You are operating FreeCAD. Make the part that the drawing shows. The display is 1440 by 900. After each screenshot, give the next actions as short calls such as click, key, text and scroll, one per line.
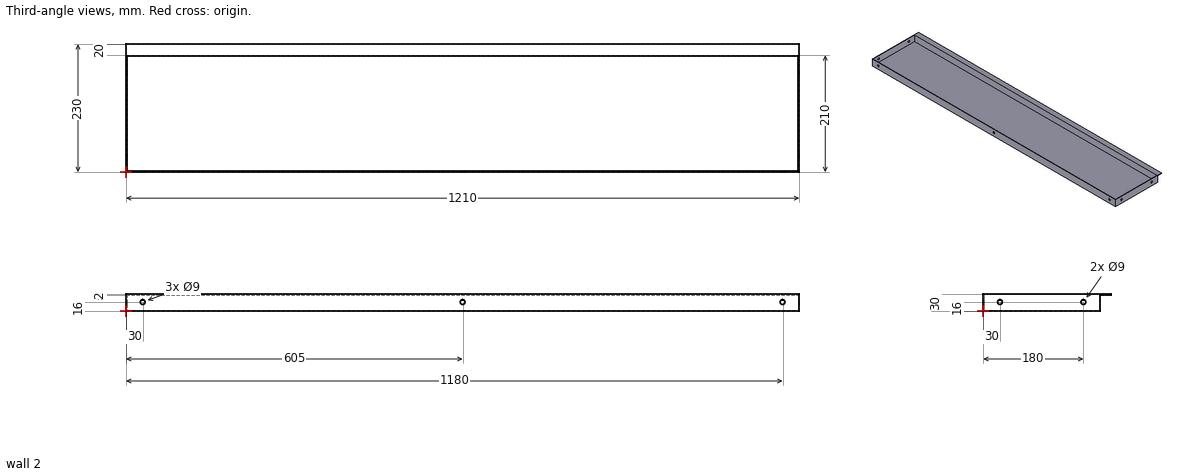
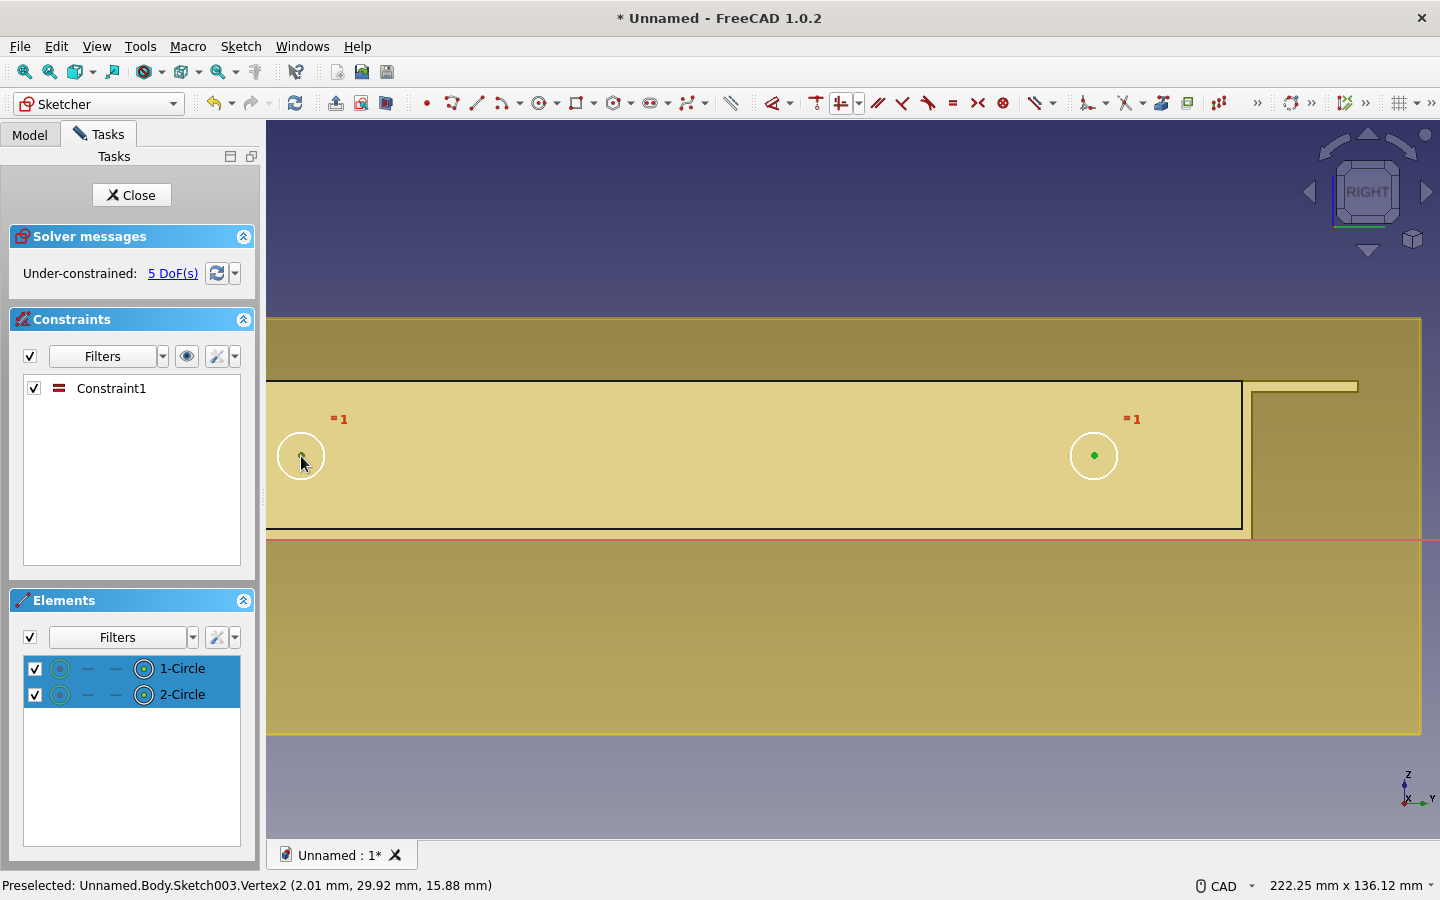
key(h)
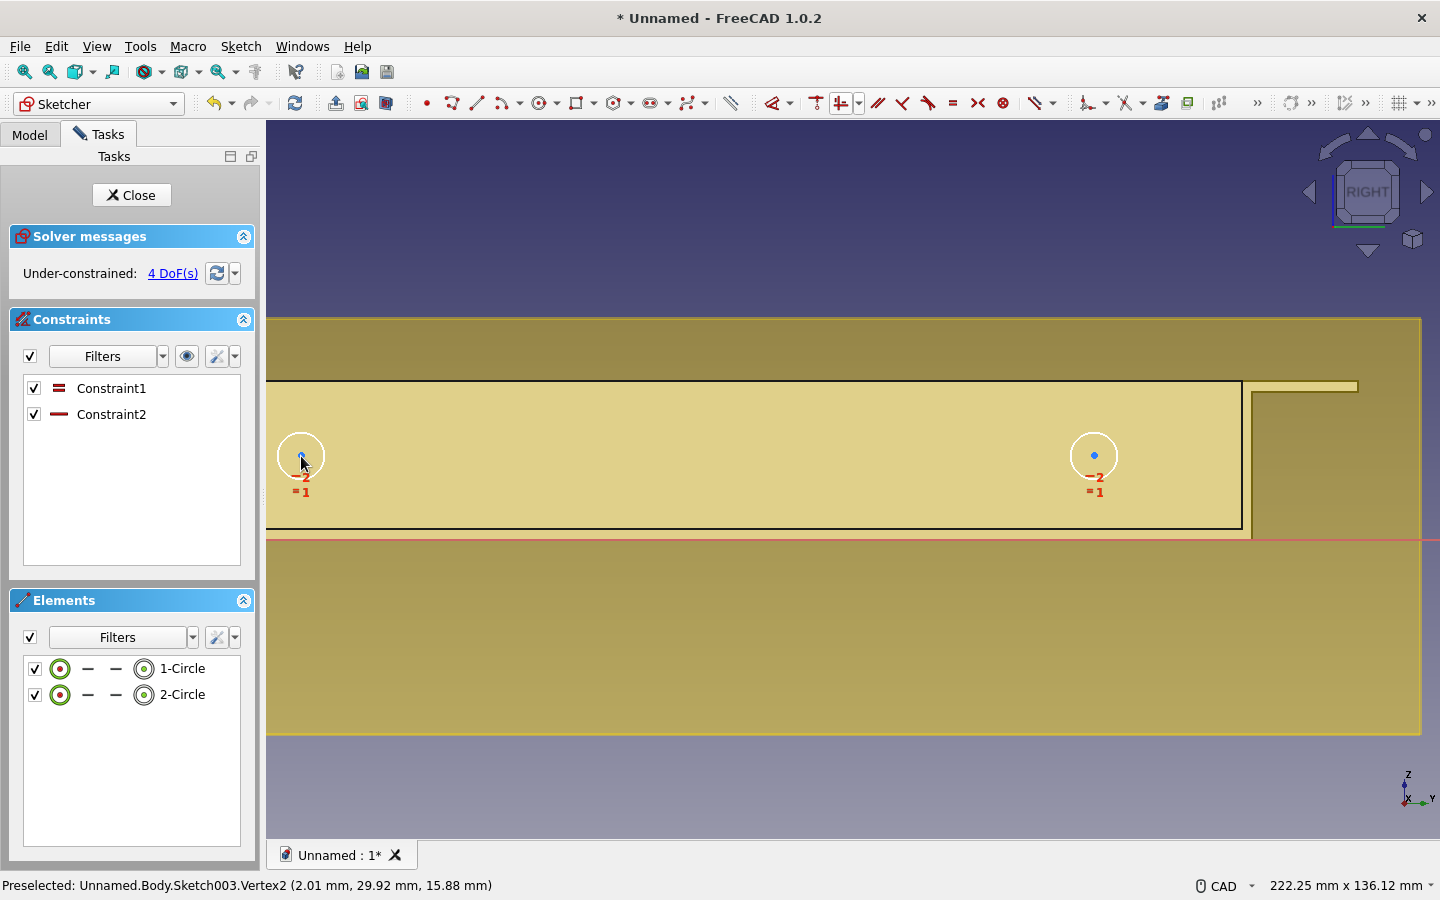
click(772, 104)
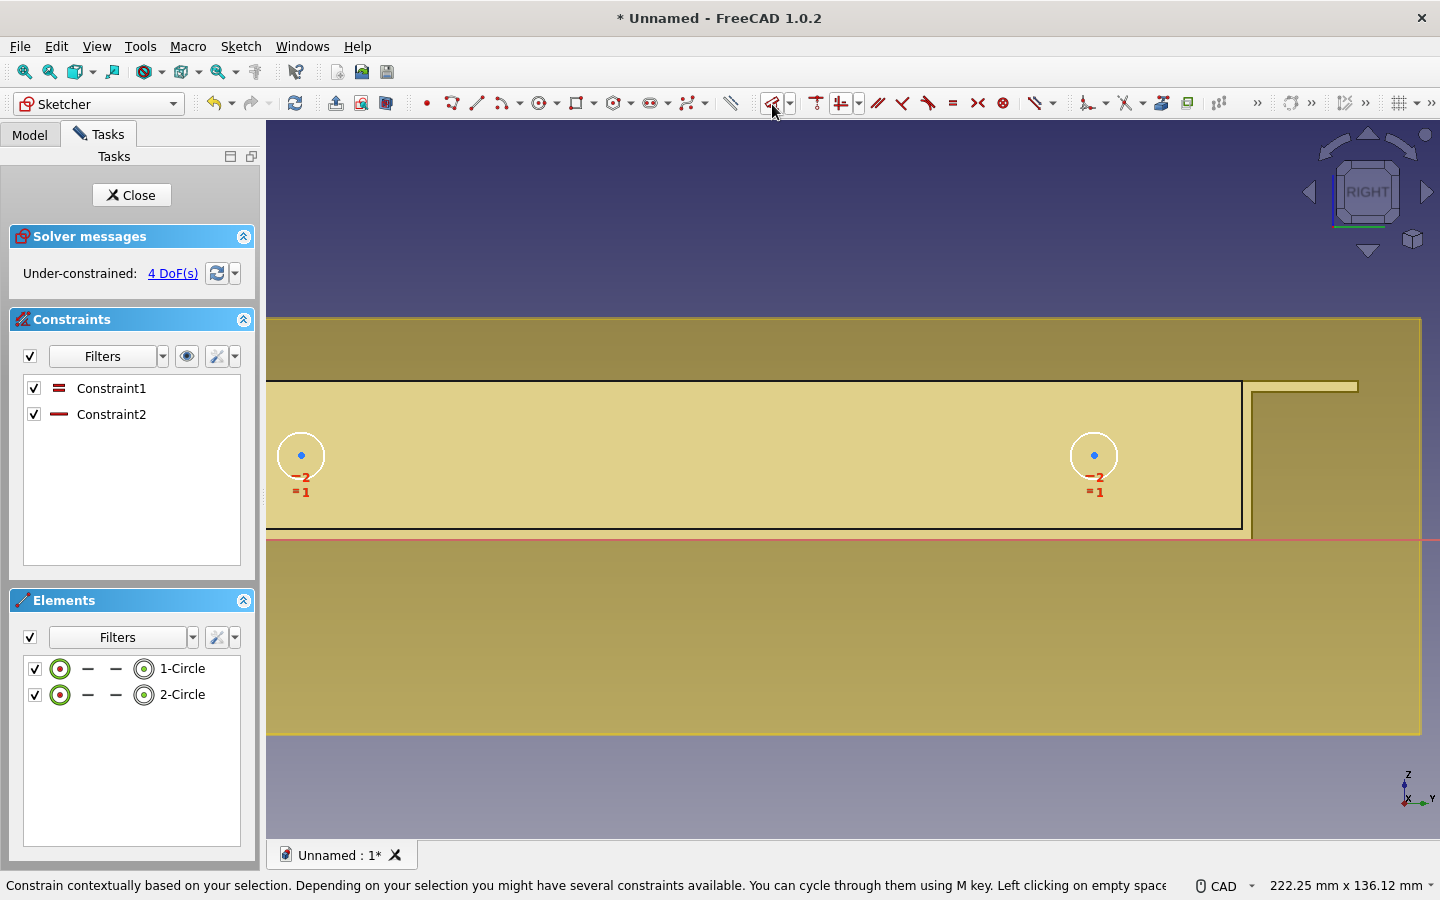
click(1110, 439)
click(1132, 416)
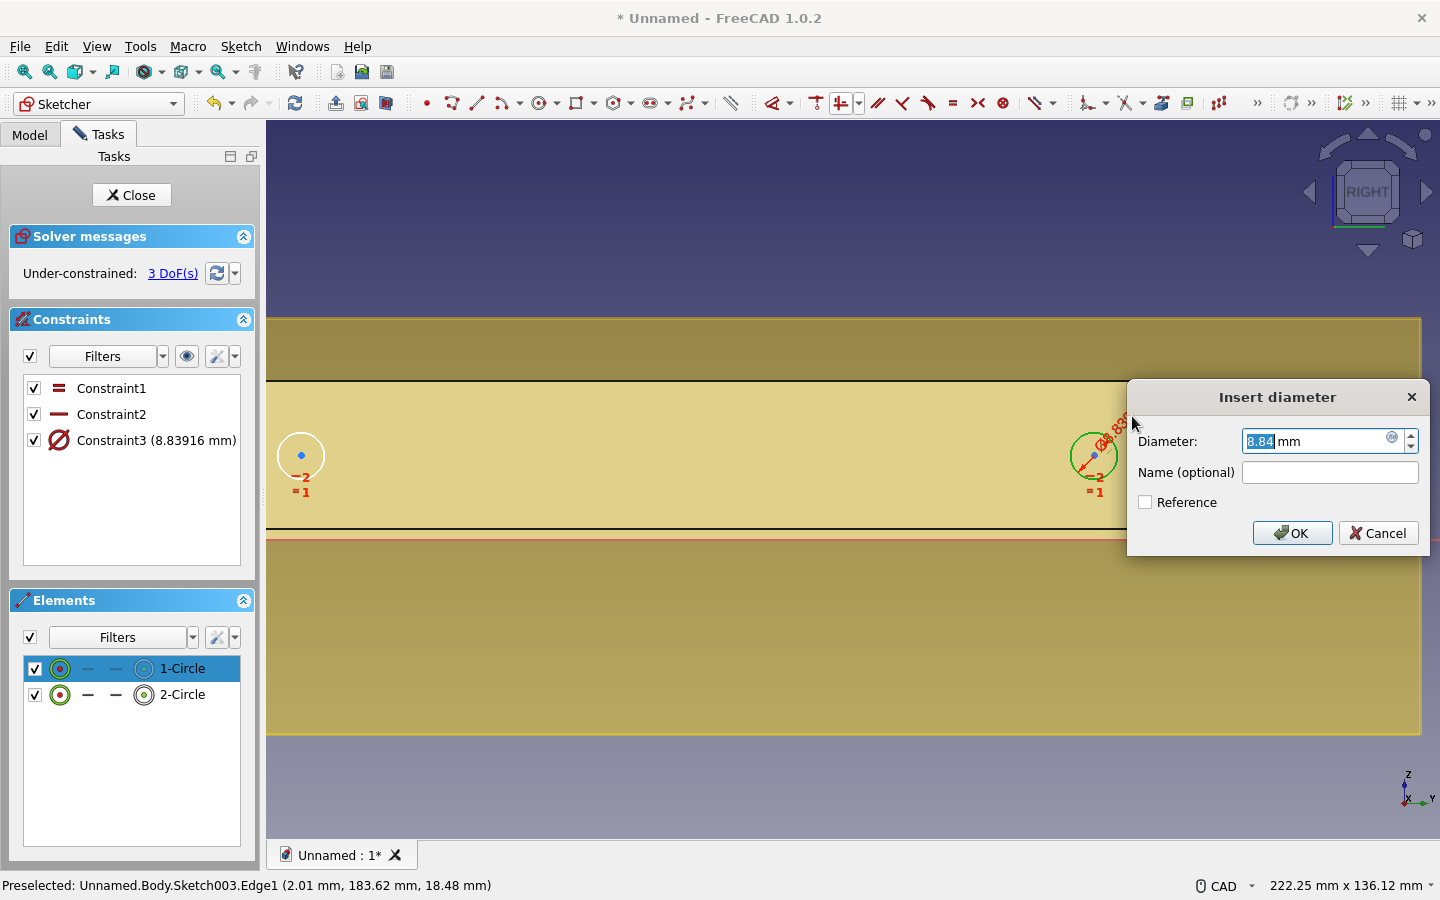
text(9)
key(Return)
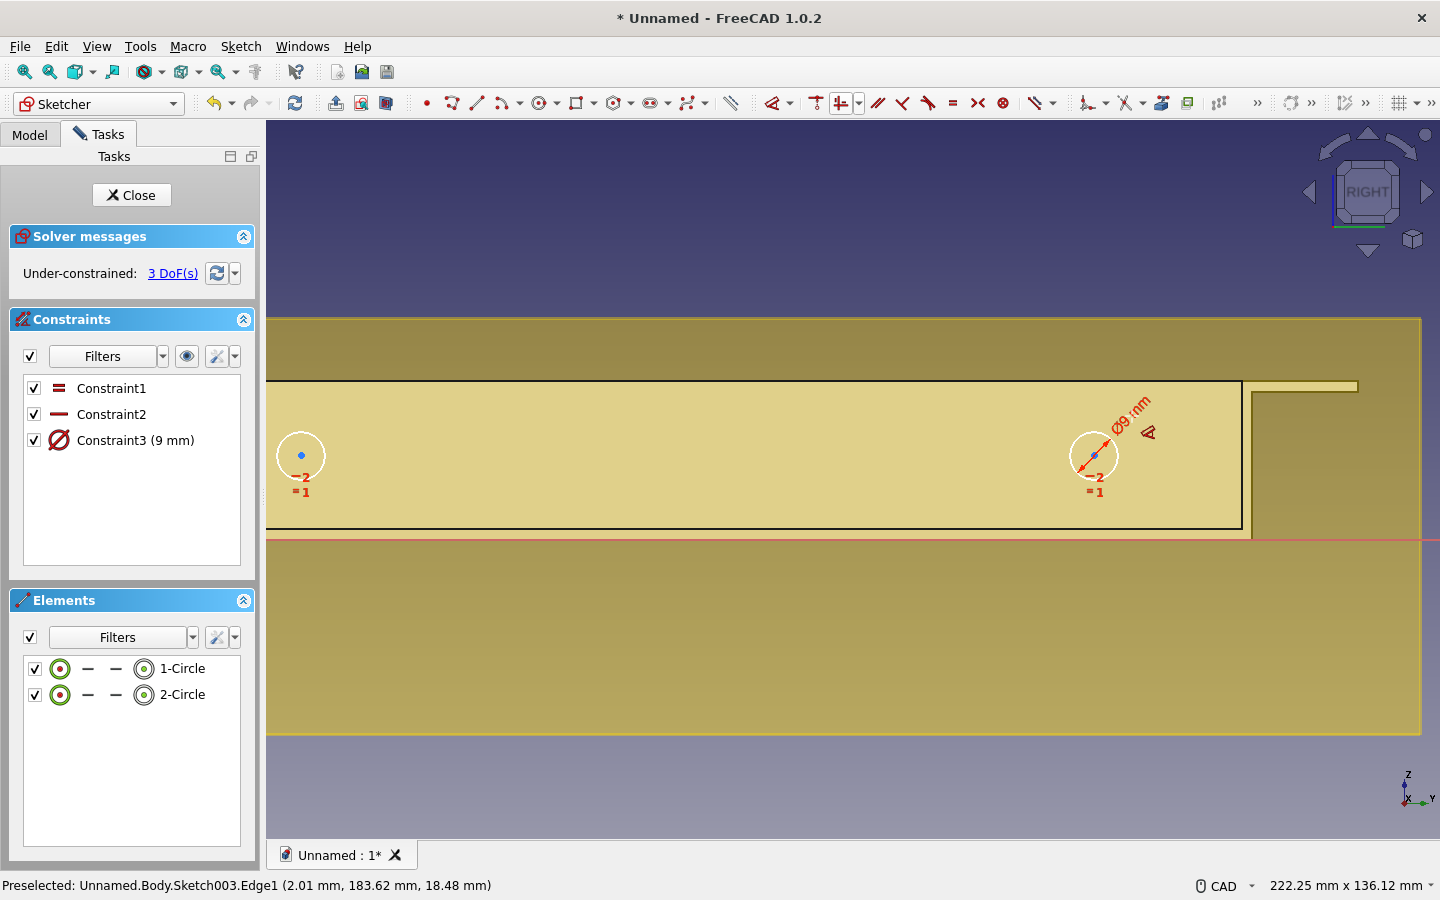
click(1094, 456)
click(1128, 498)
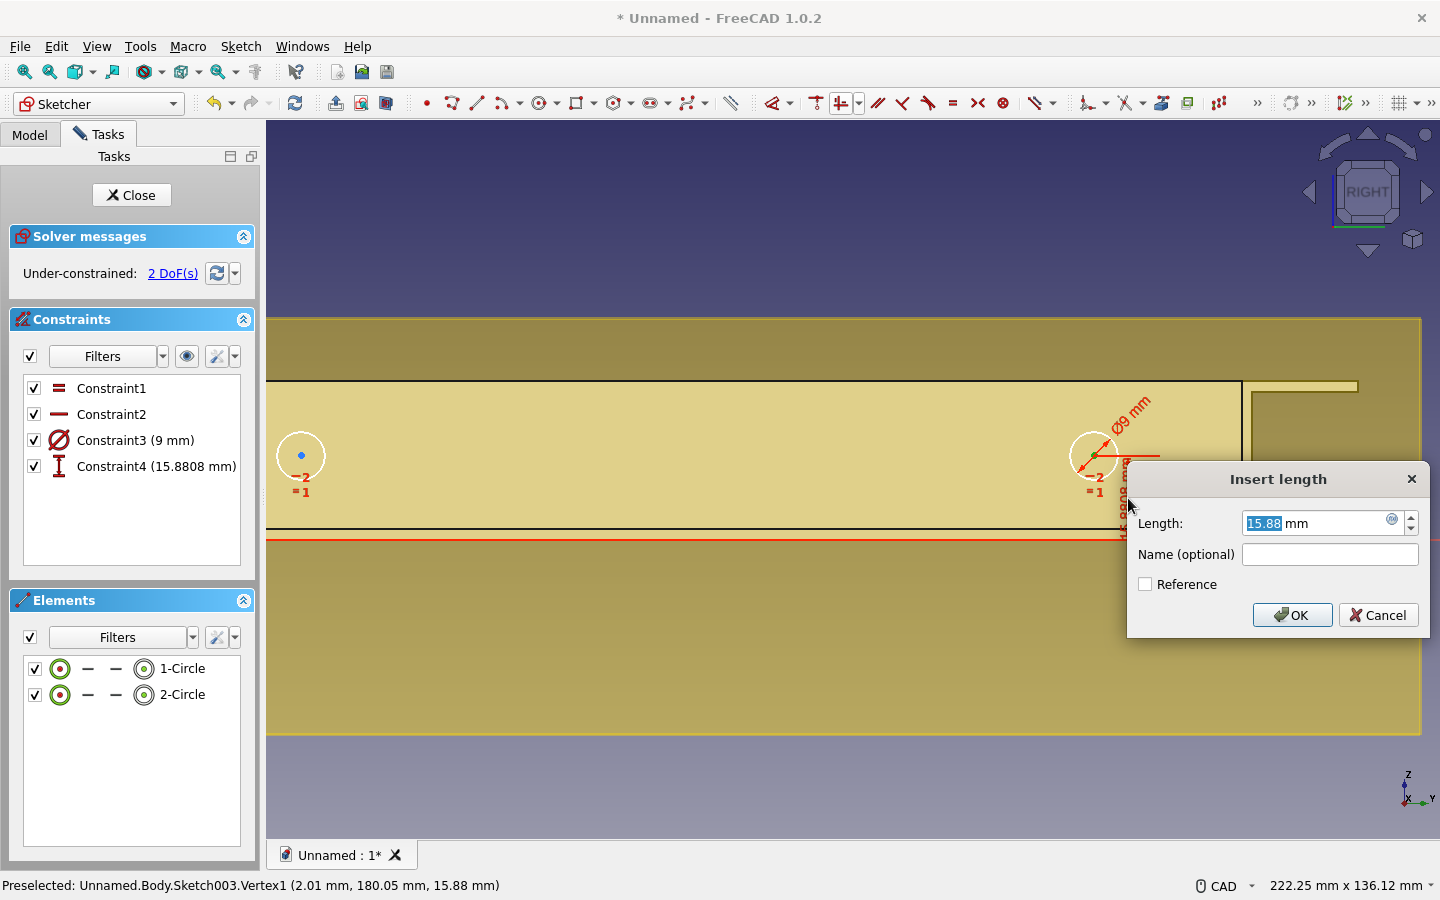
text(16)
key(Return)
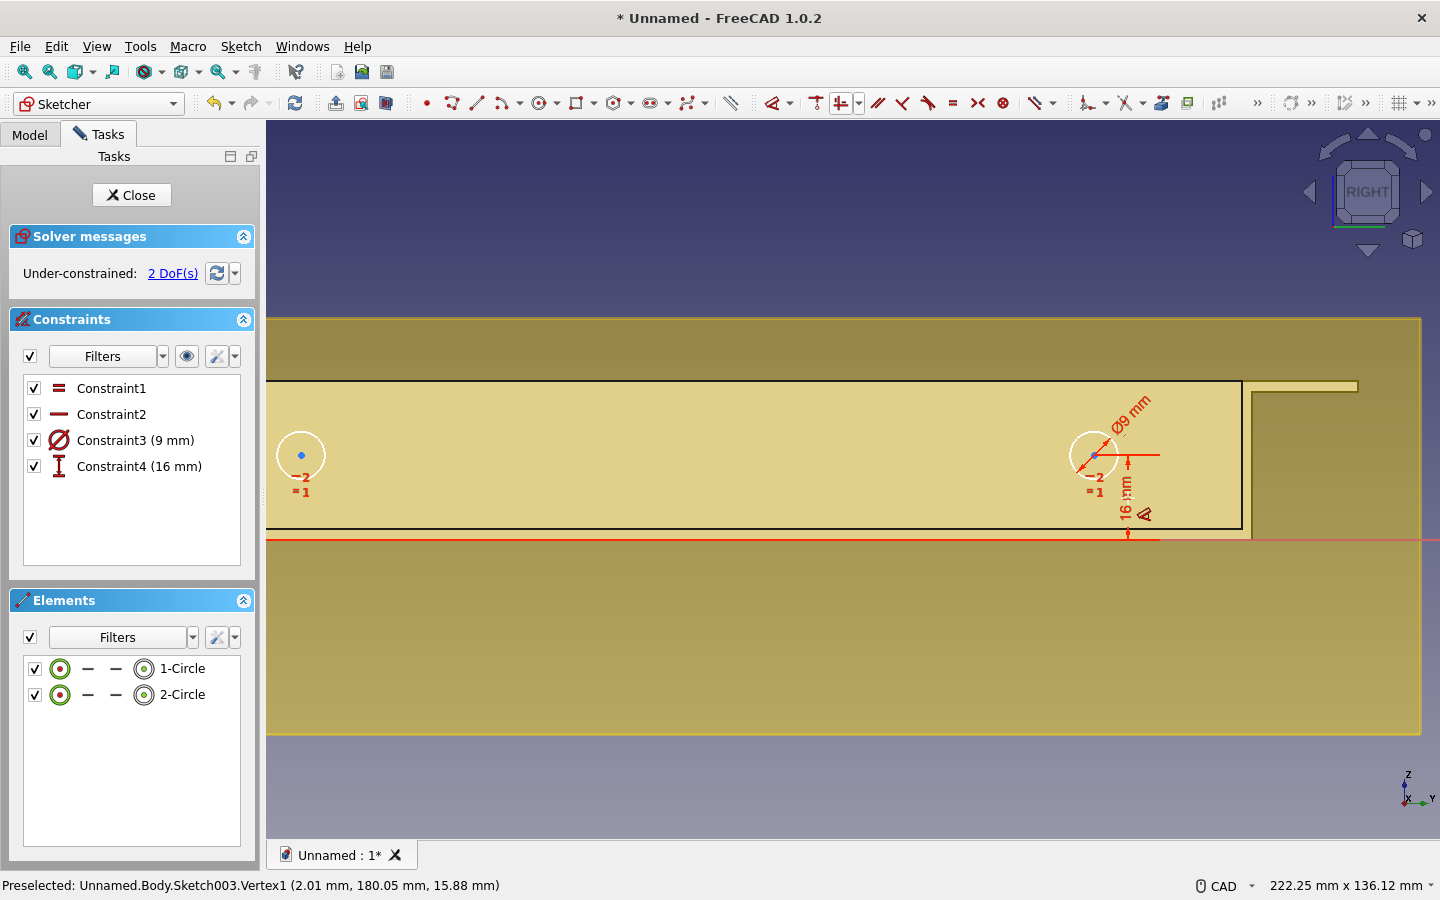
click(301, 455)
click(297, 574)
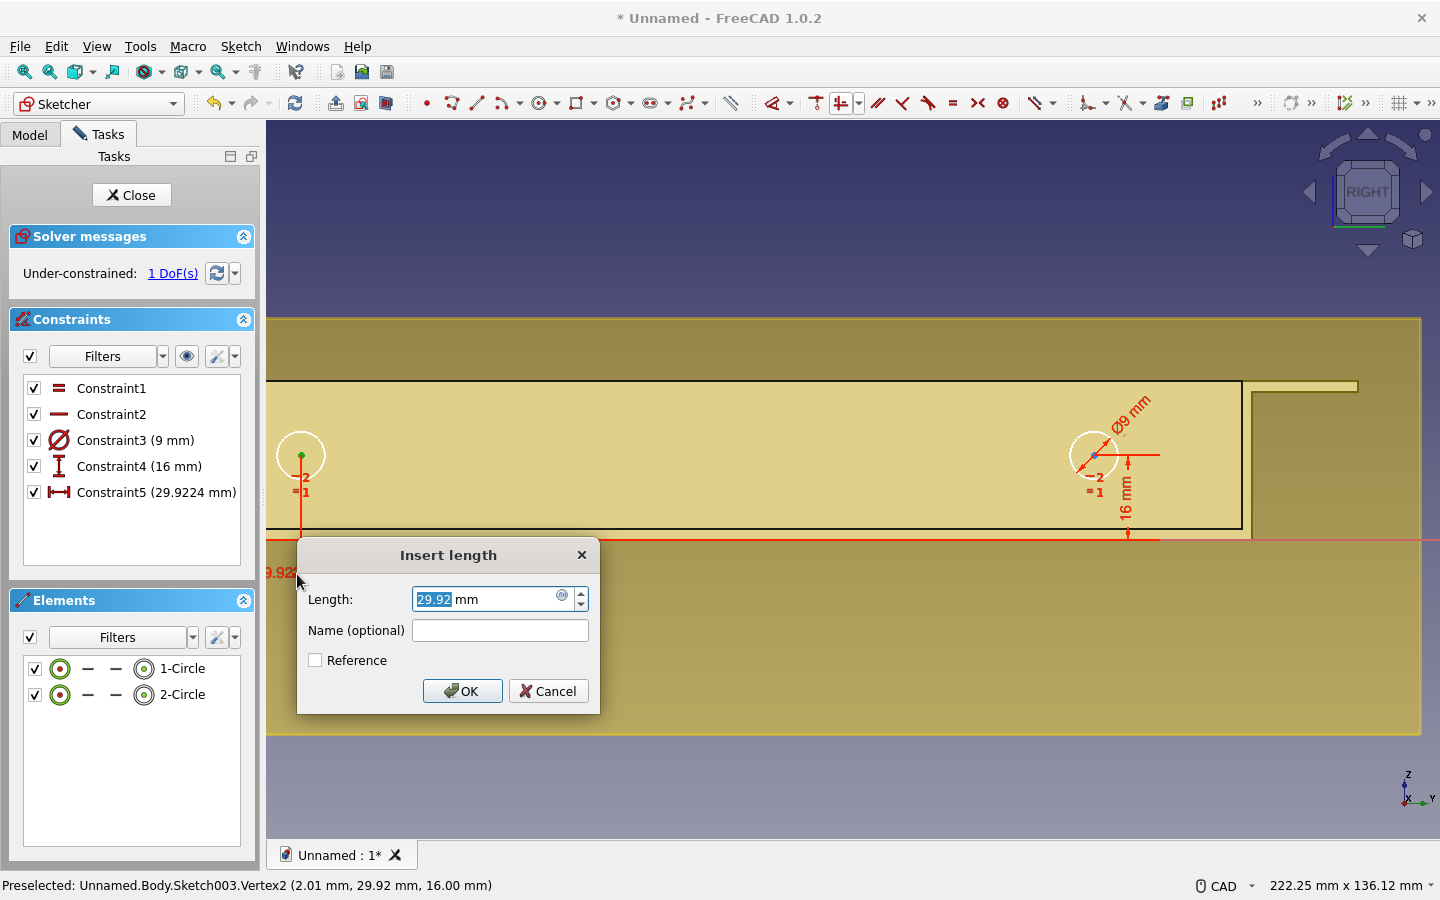
text(30)
key(Return)